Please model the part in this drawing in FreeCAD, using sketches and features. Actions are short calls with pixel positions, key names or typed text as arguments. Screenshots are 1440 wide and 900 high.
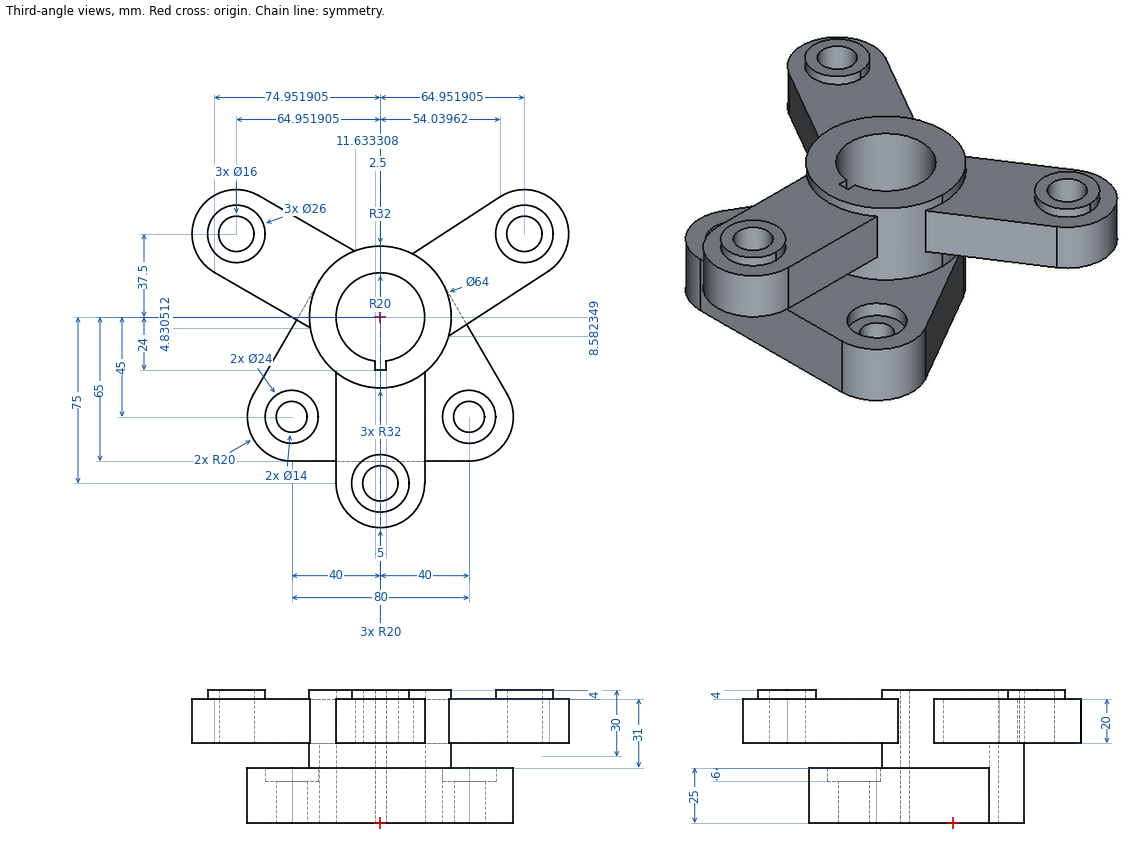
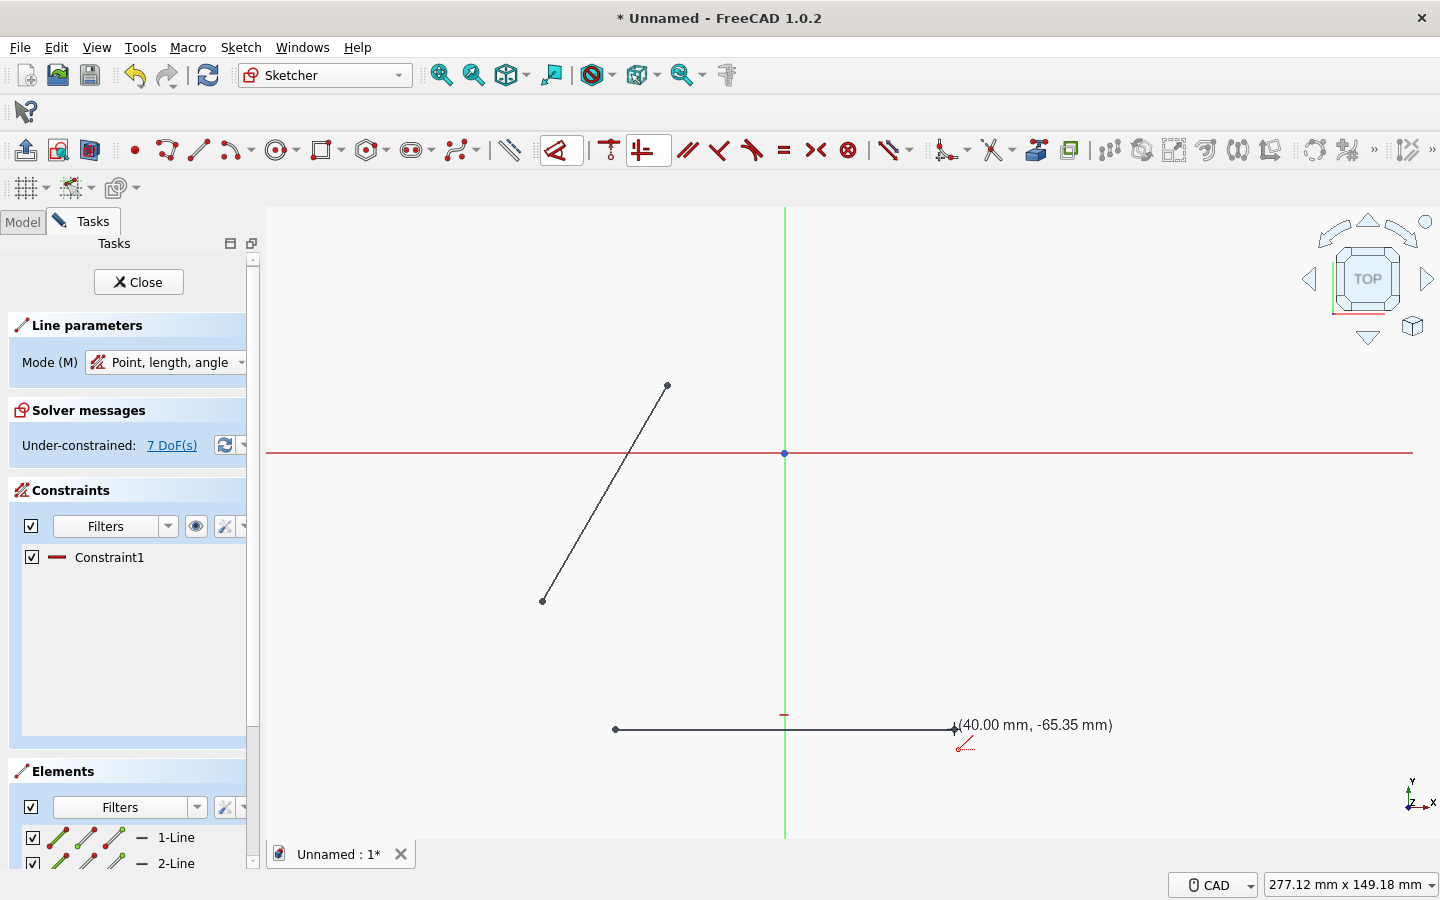
click(1027, 601)
click(902, 385)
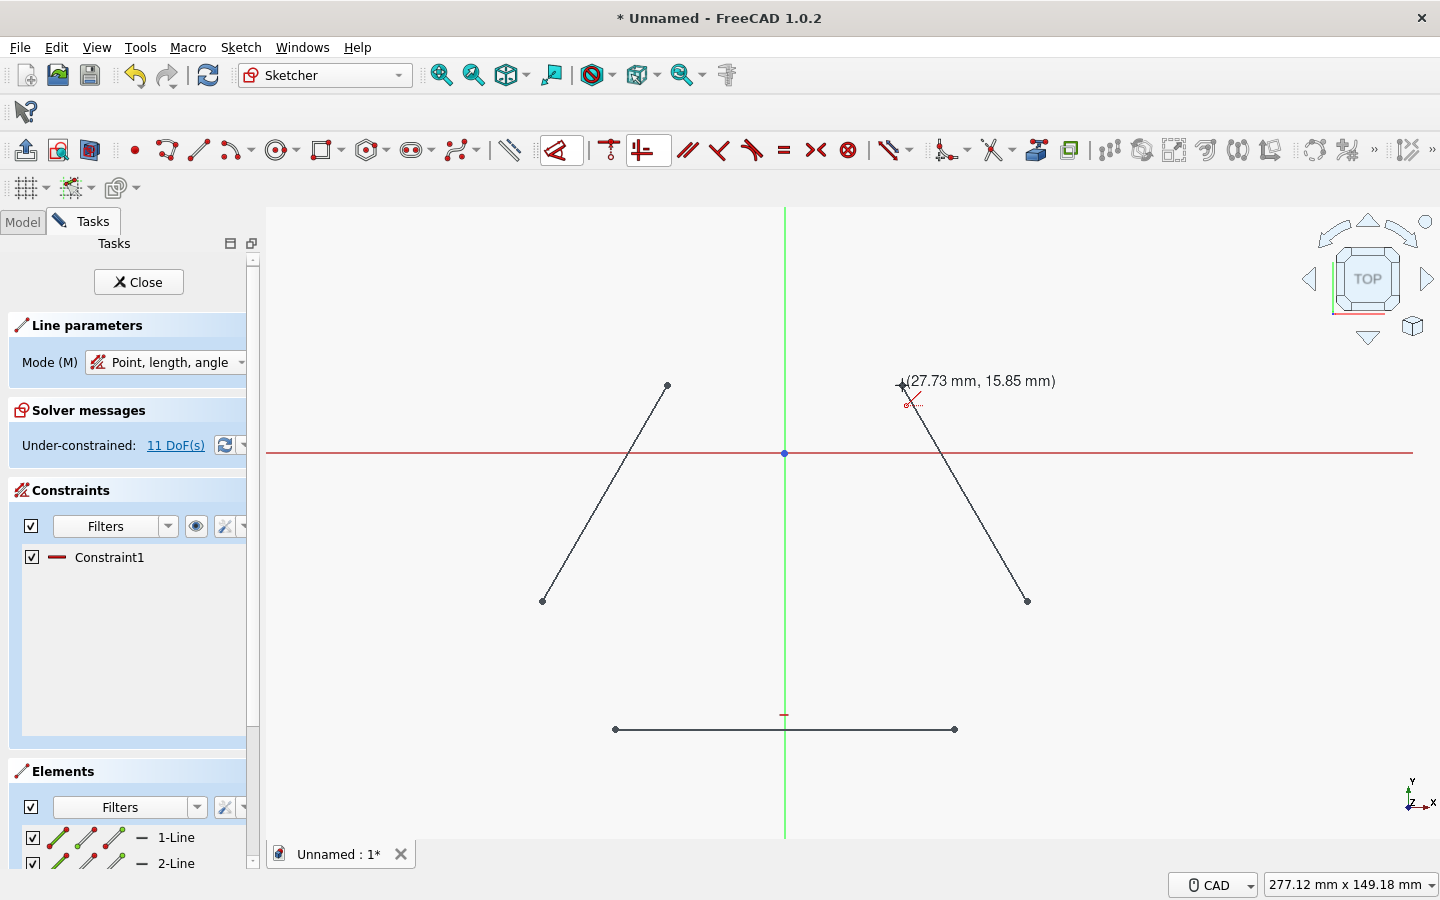
key(g)
key(3)
key(a)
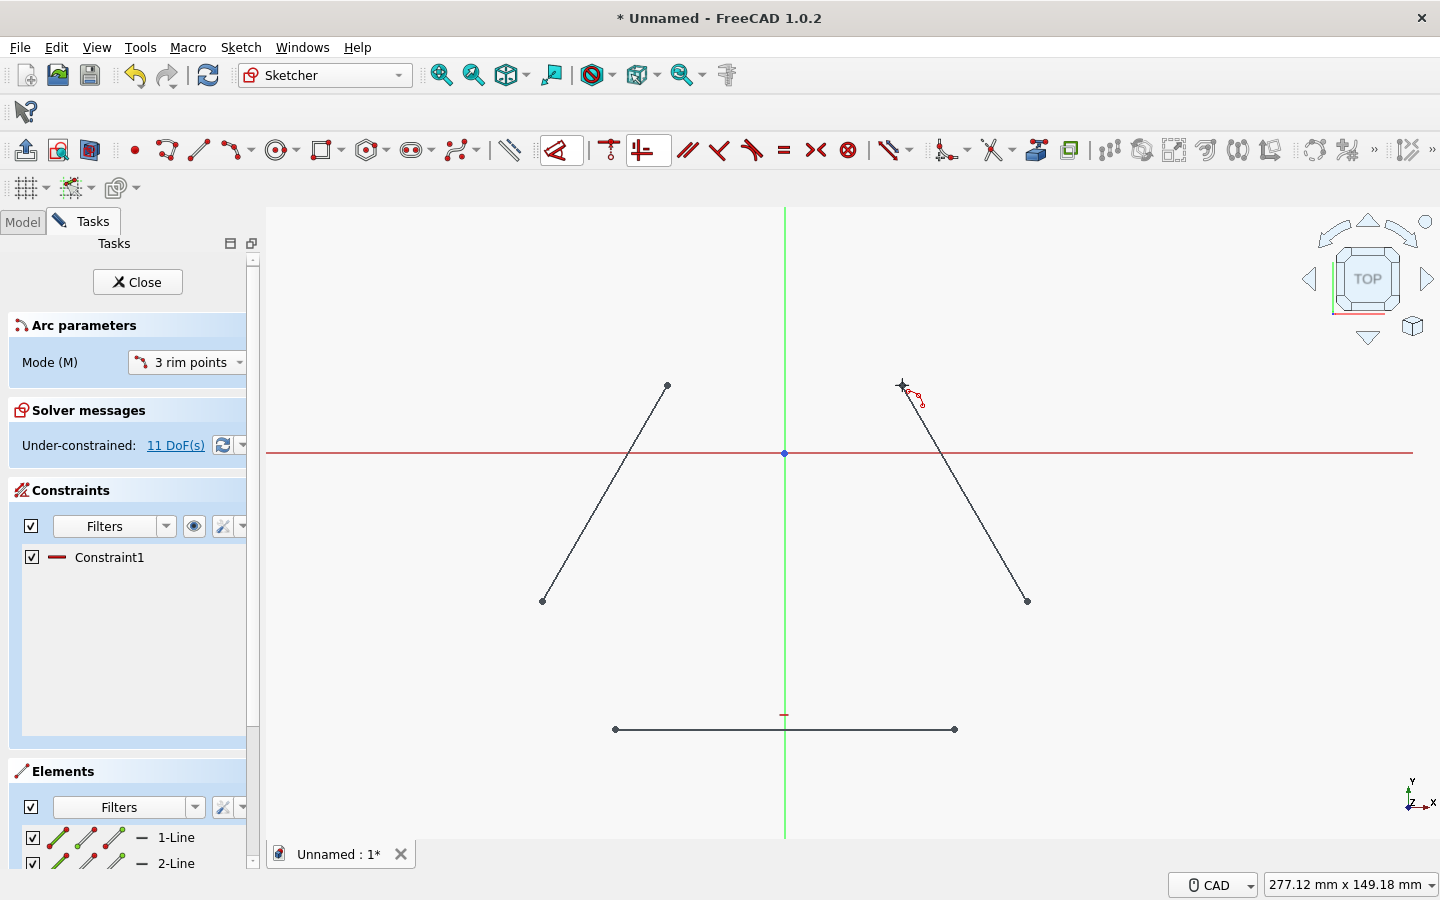
click(542, 602)
click(615, 730)
click(542, 686)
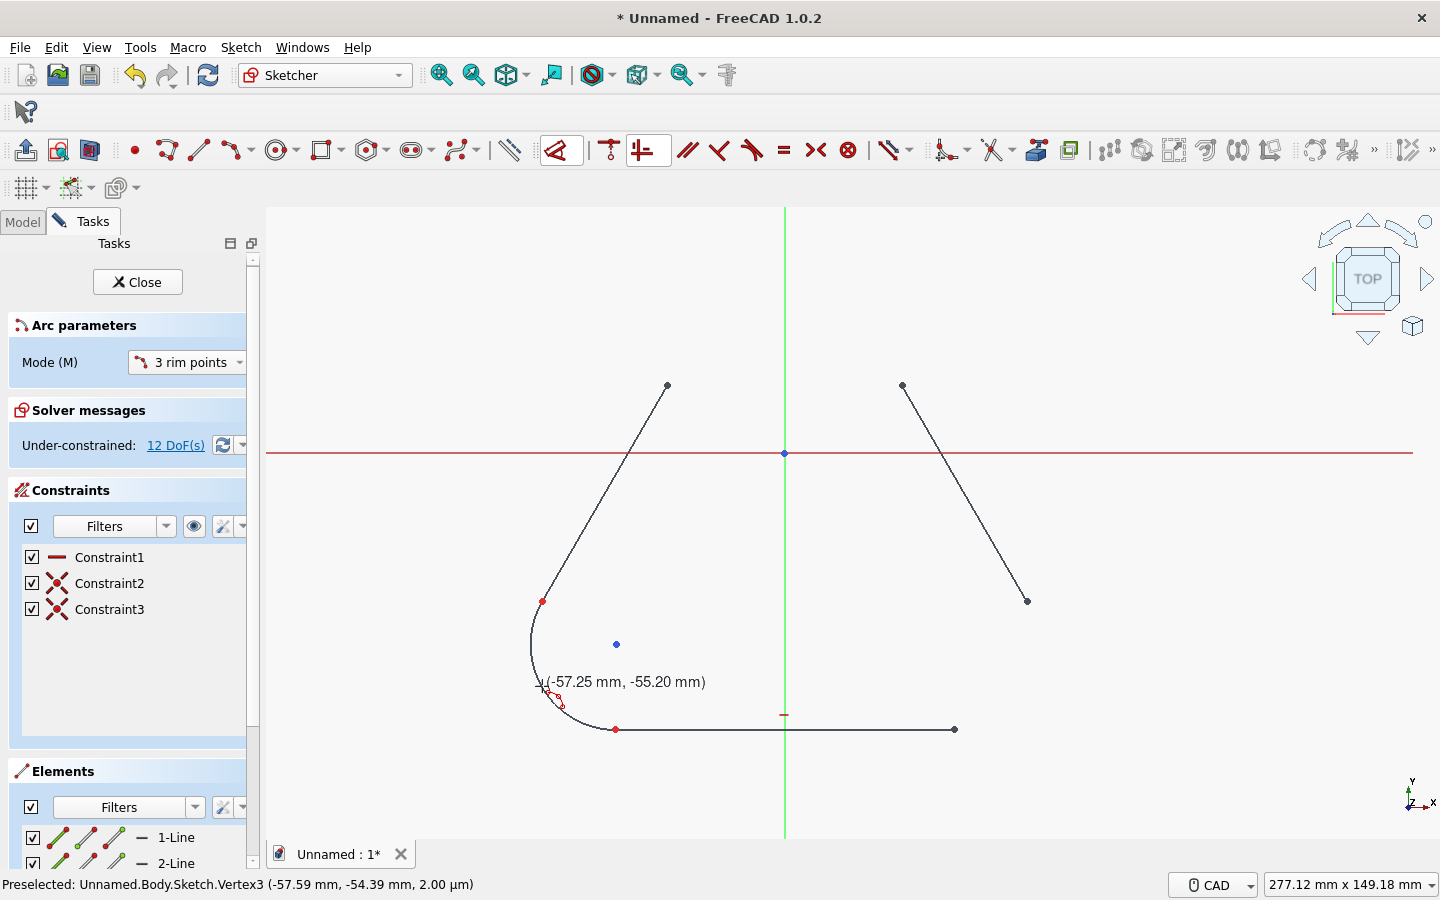
click(954, 730)
click(1027, 602)
click(1027, 686)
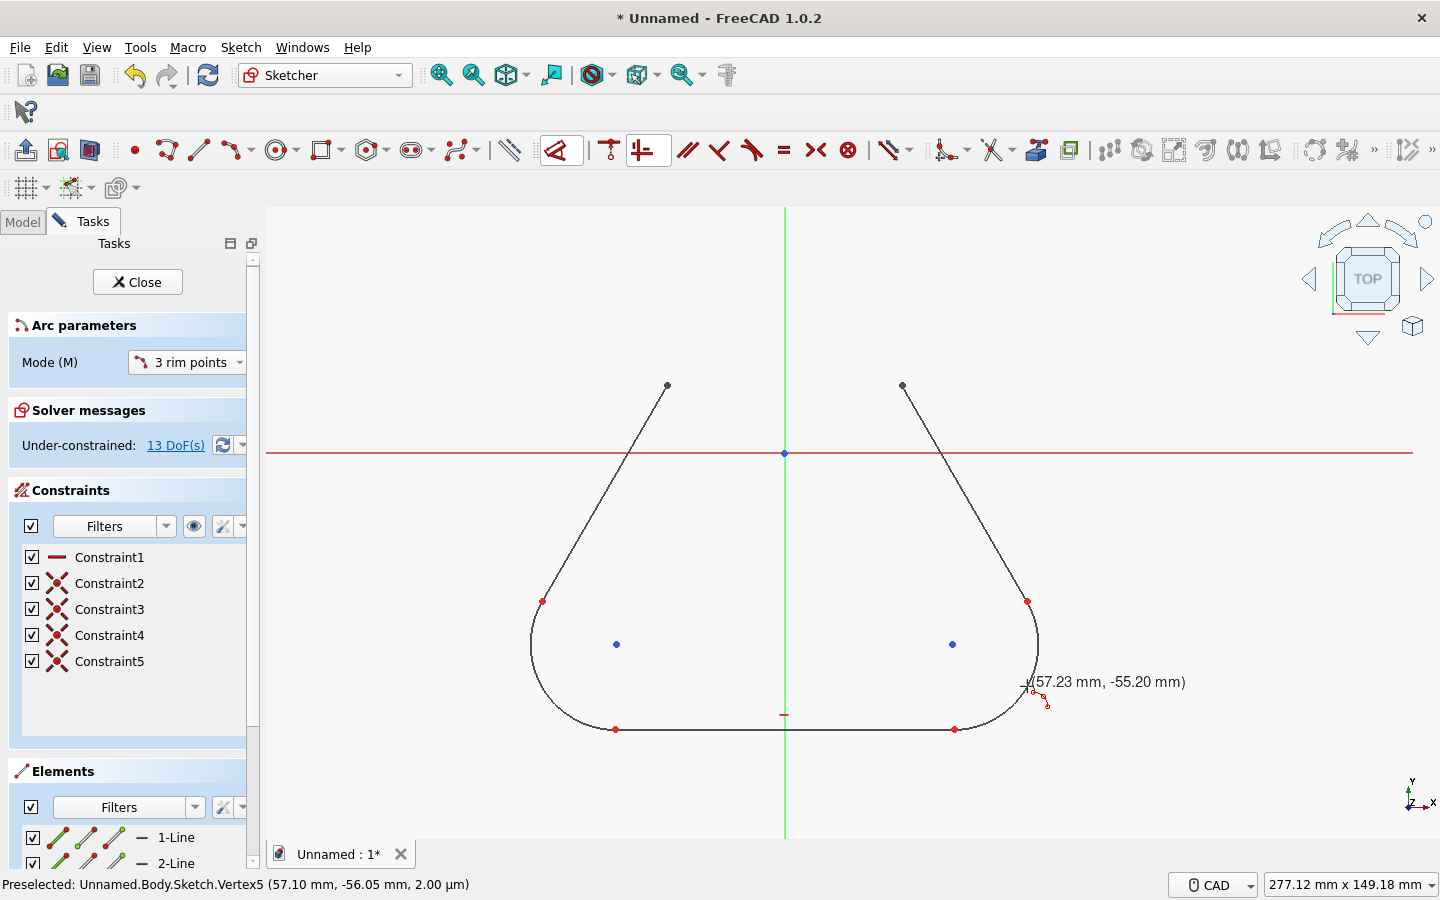
click(902, 386)
click(667, 386)
click(813, 321)
key(Escape)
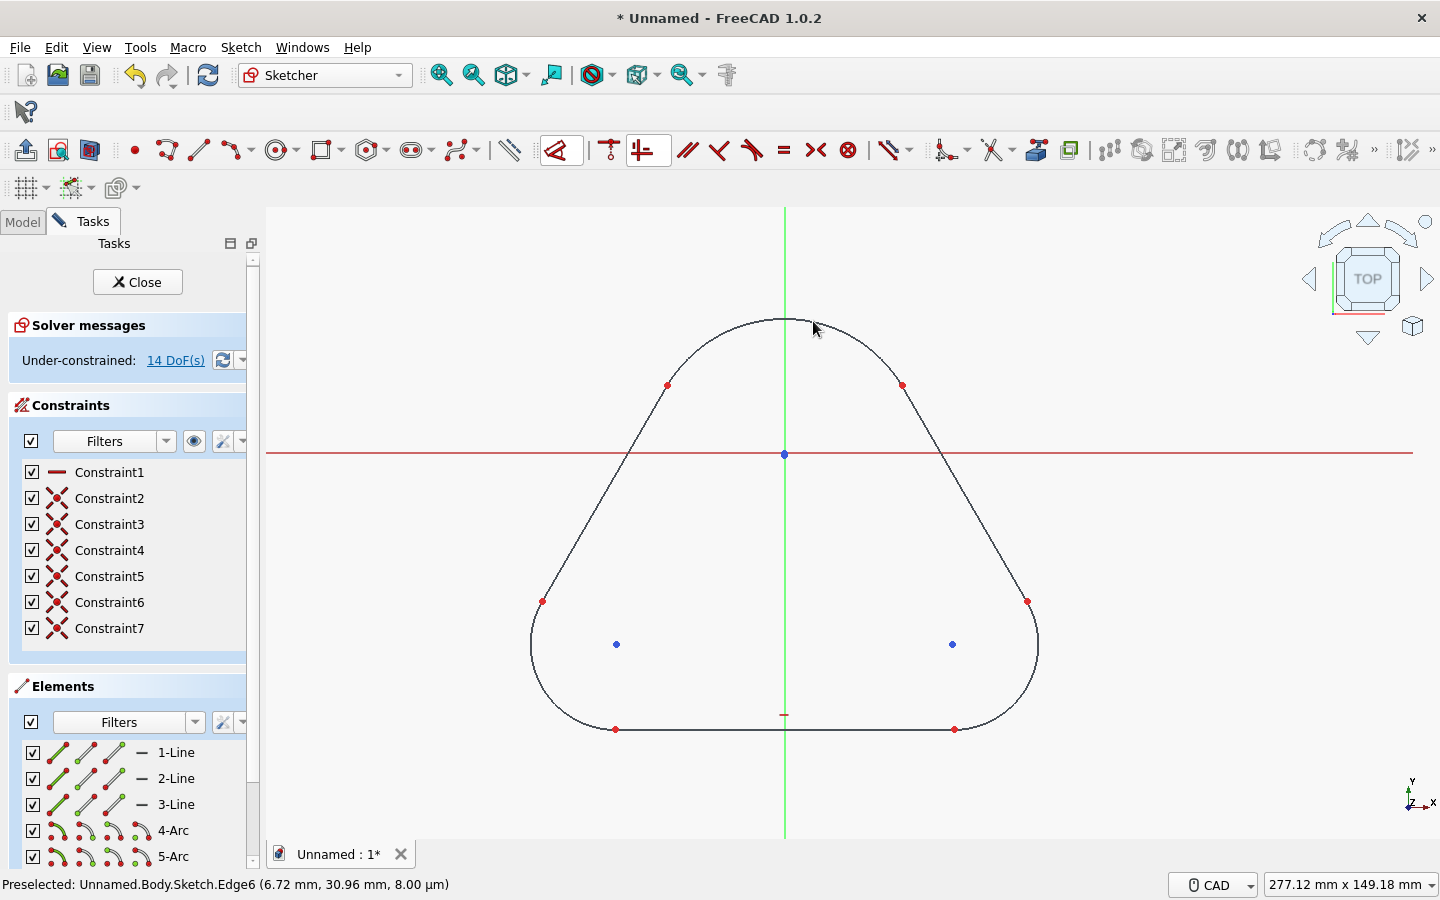
click(629, 451)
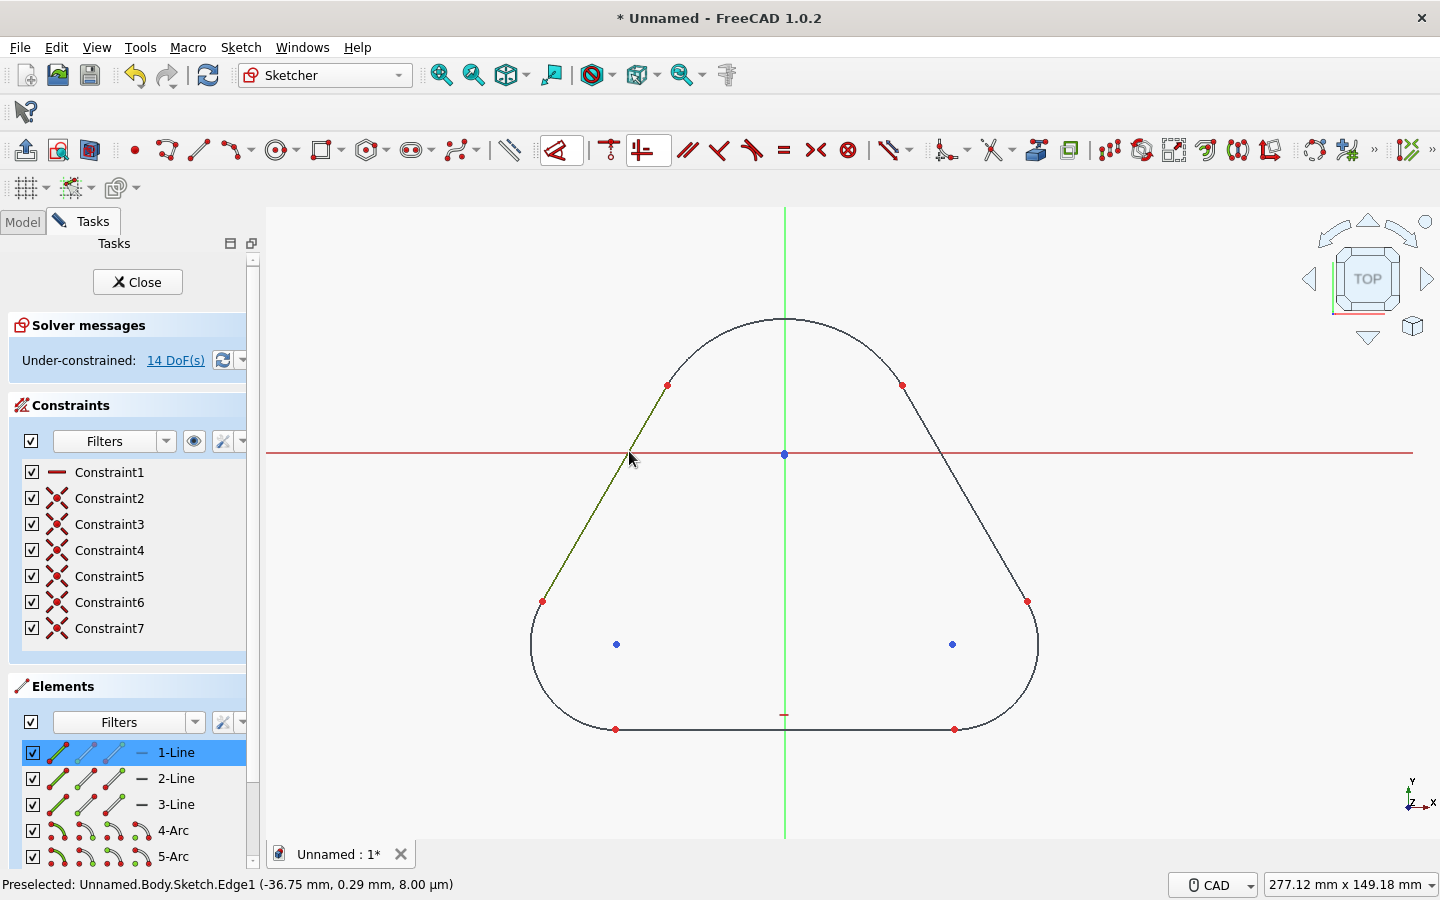
click(531, 653)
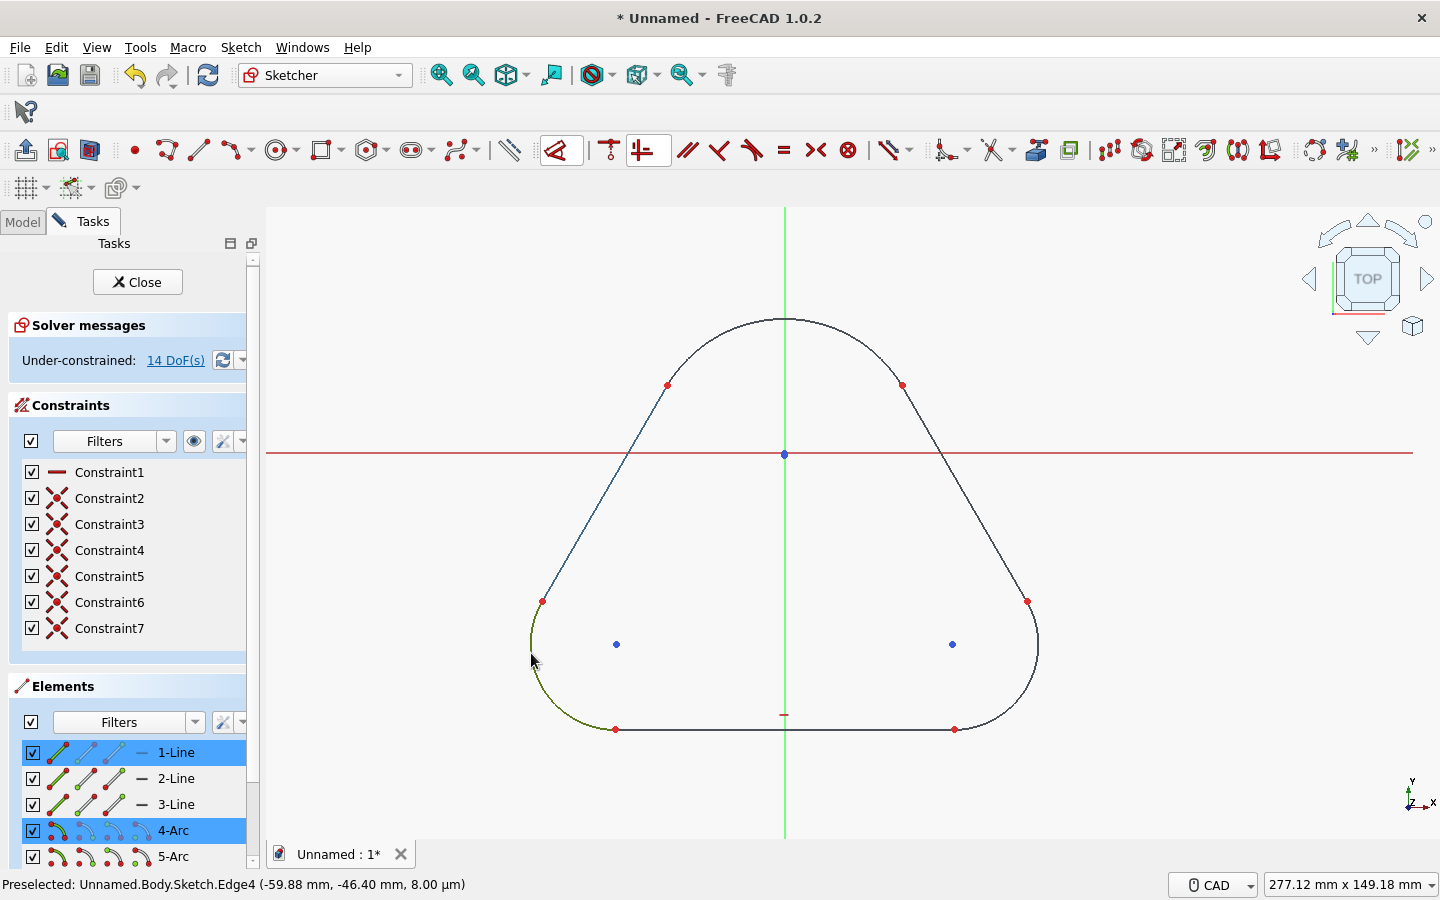
click(752, 150)